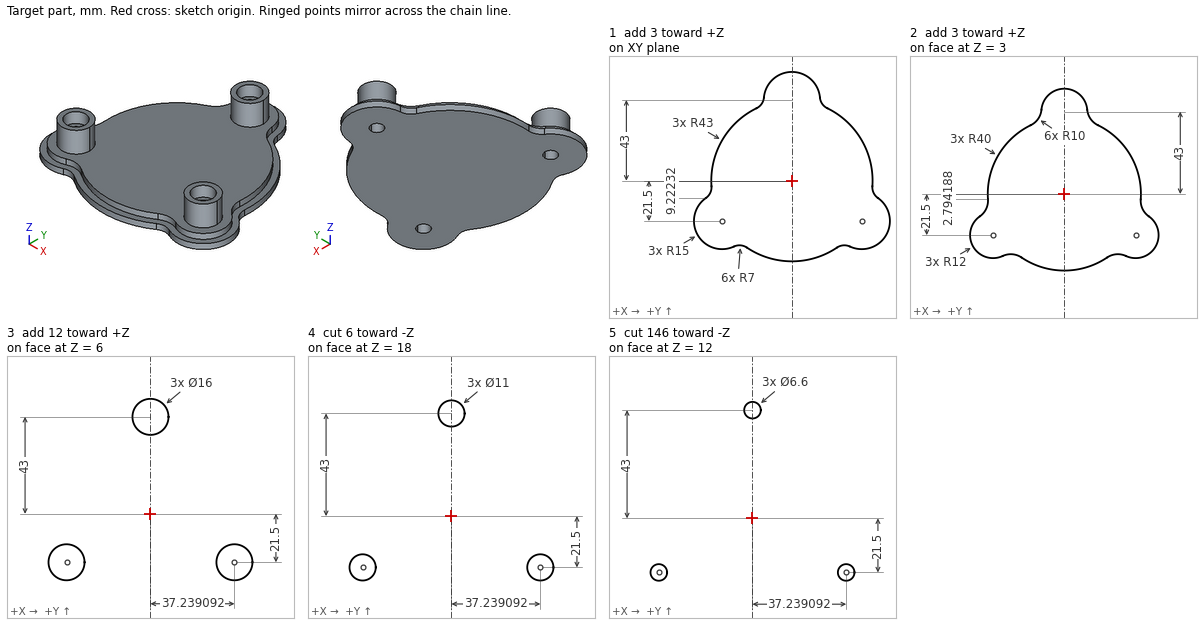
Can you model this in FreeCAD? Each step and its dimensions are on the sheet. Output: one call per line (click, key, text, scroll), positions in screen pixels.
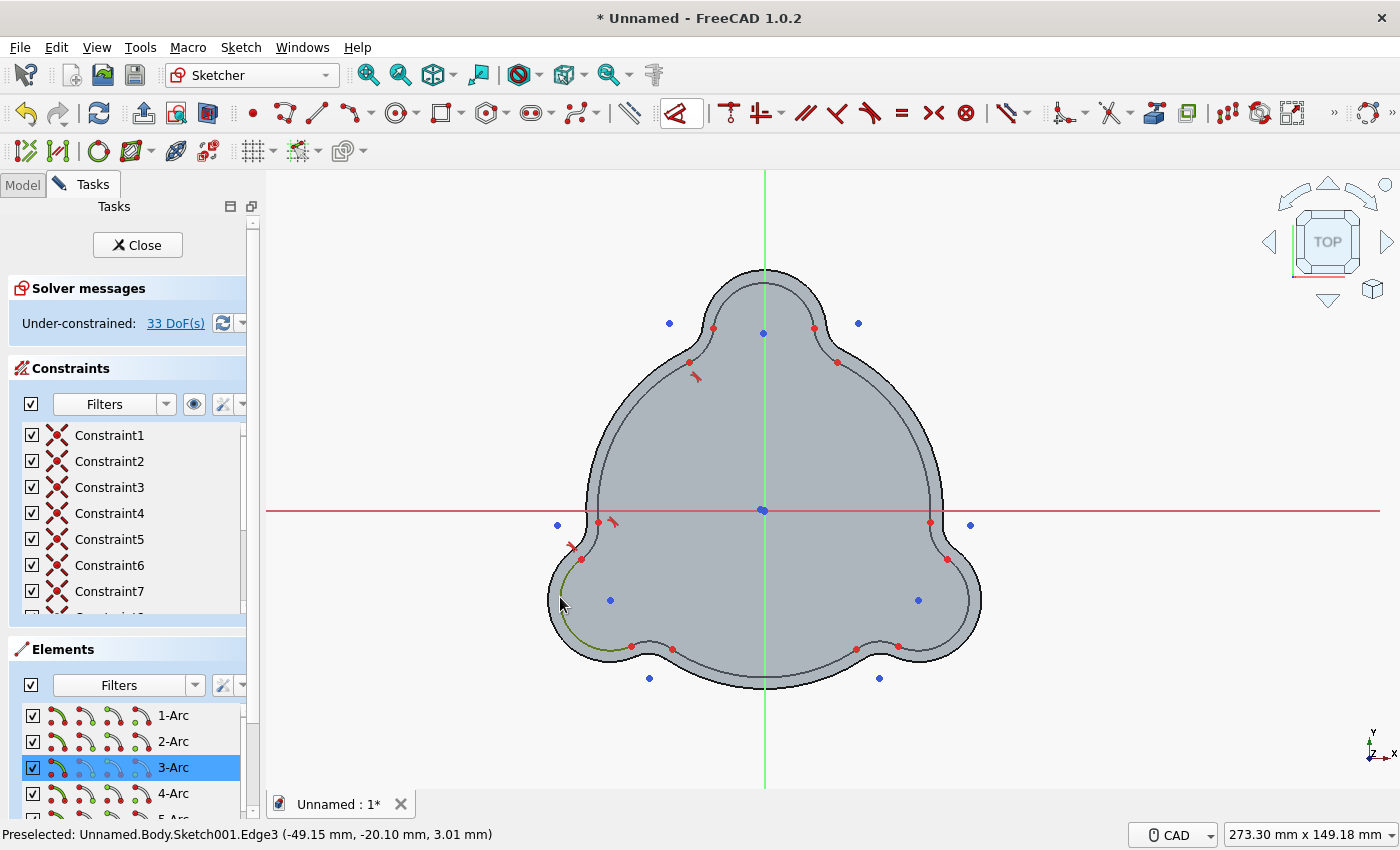
click(661, 643)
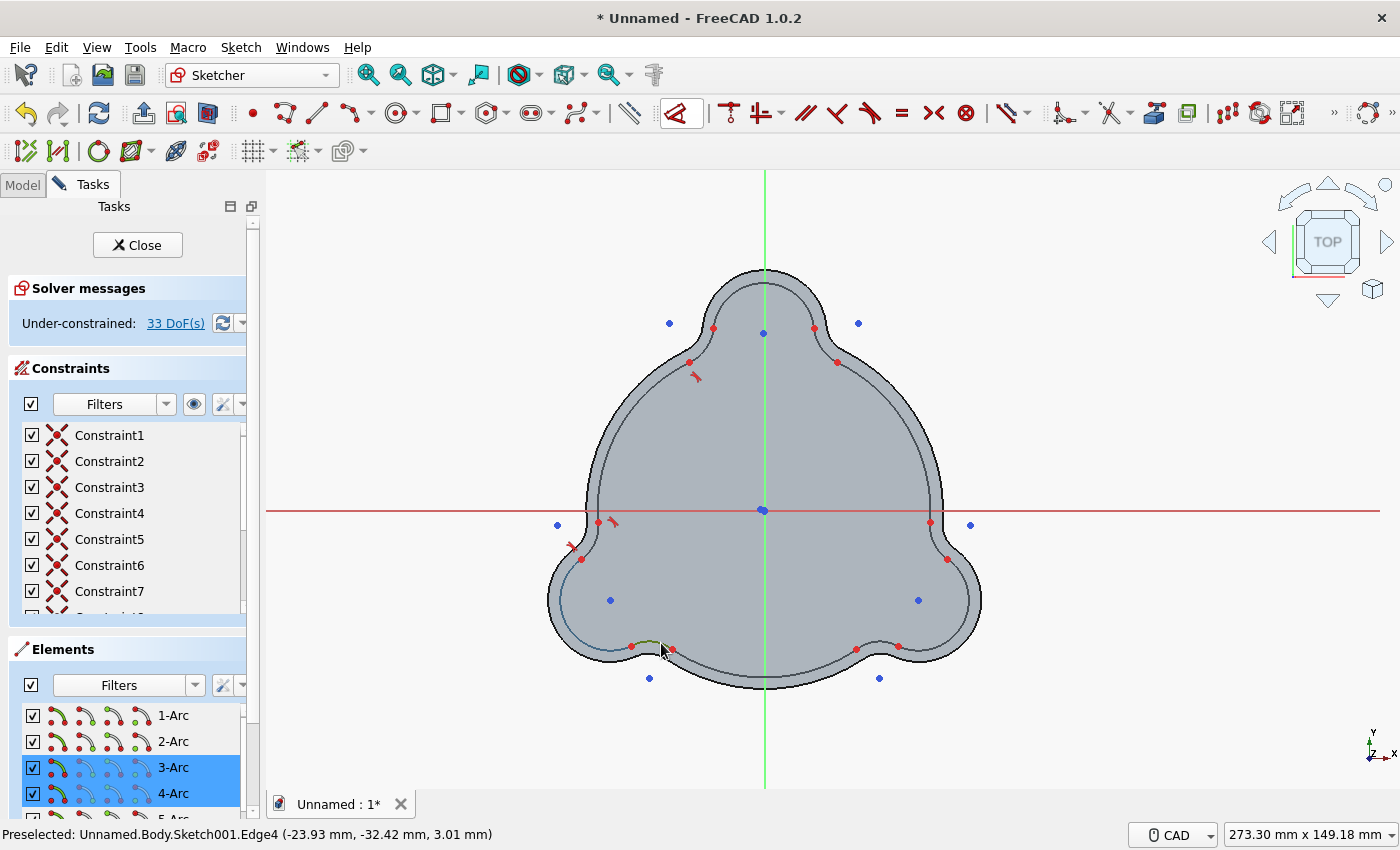
click(870, 114)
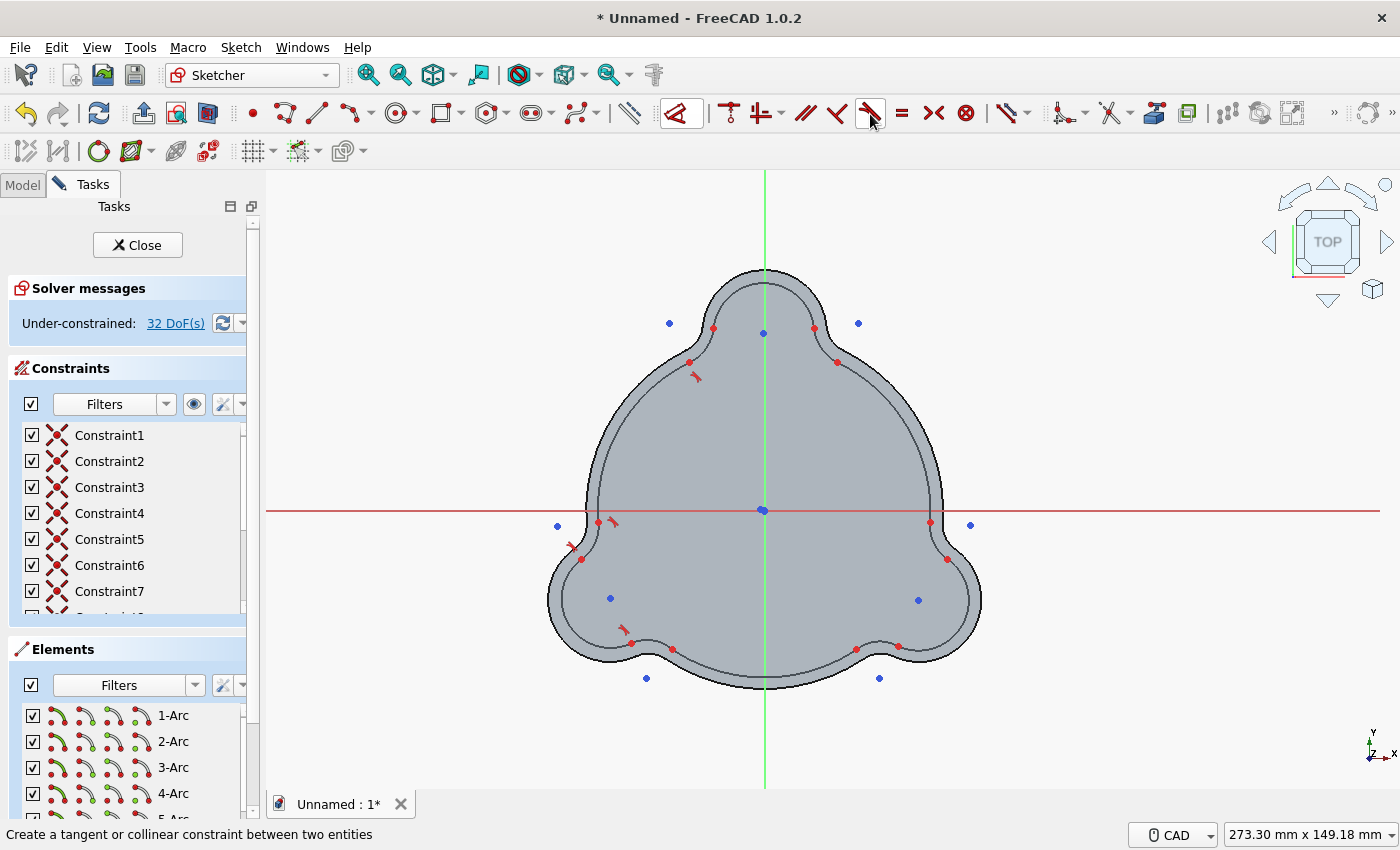
click(661, 643)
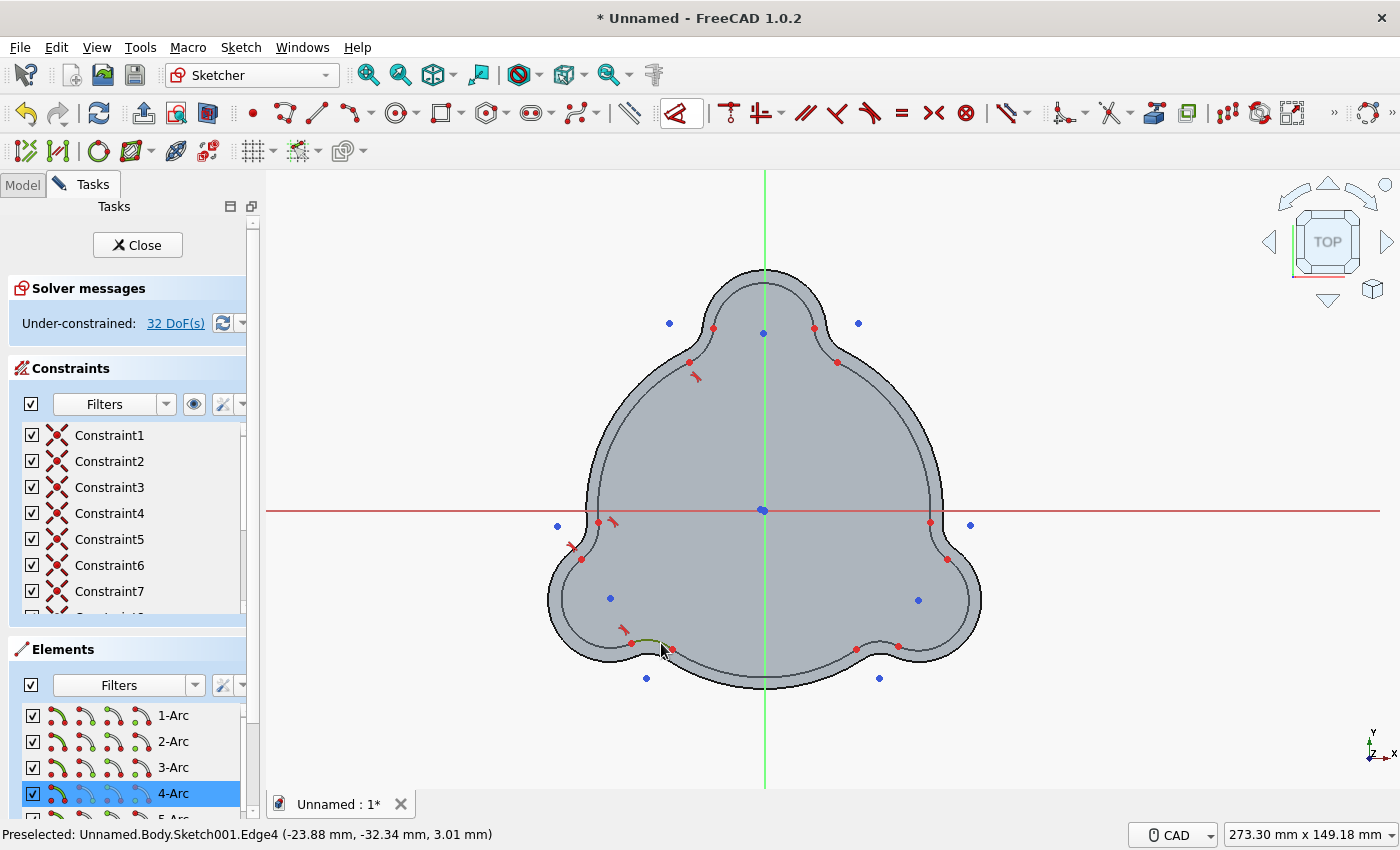
click(726, 673)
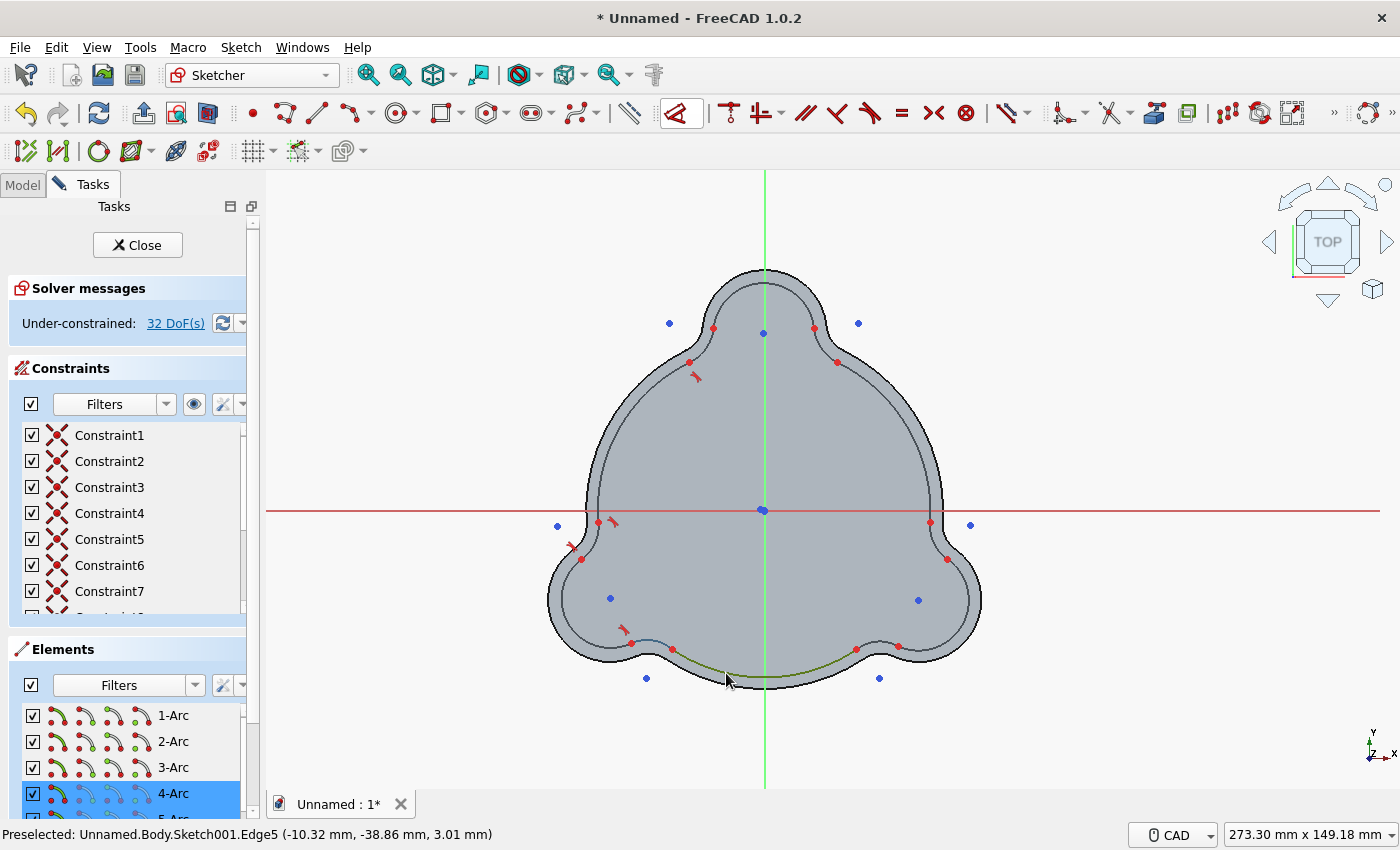
click(870, 114)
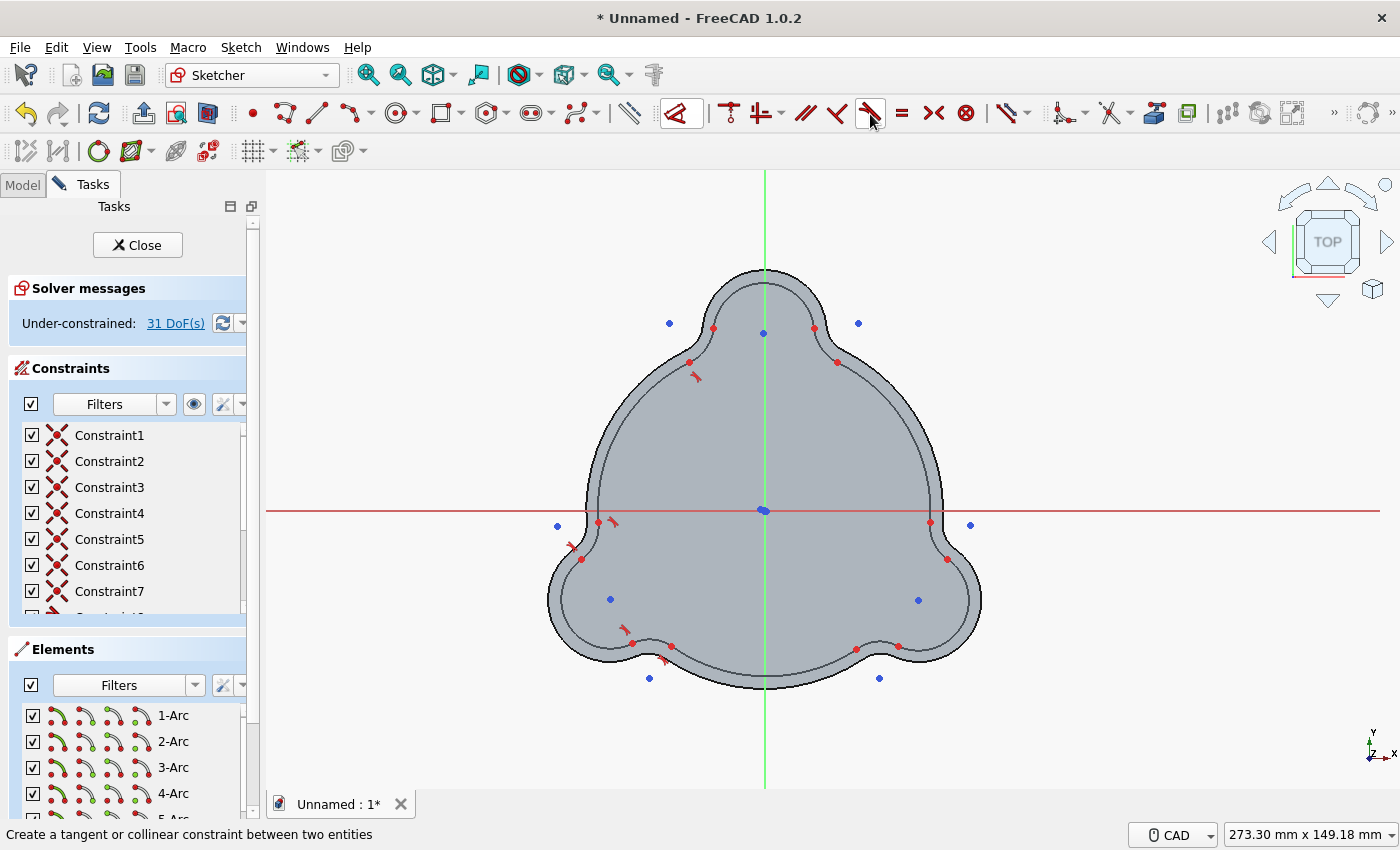
click(725, 671)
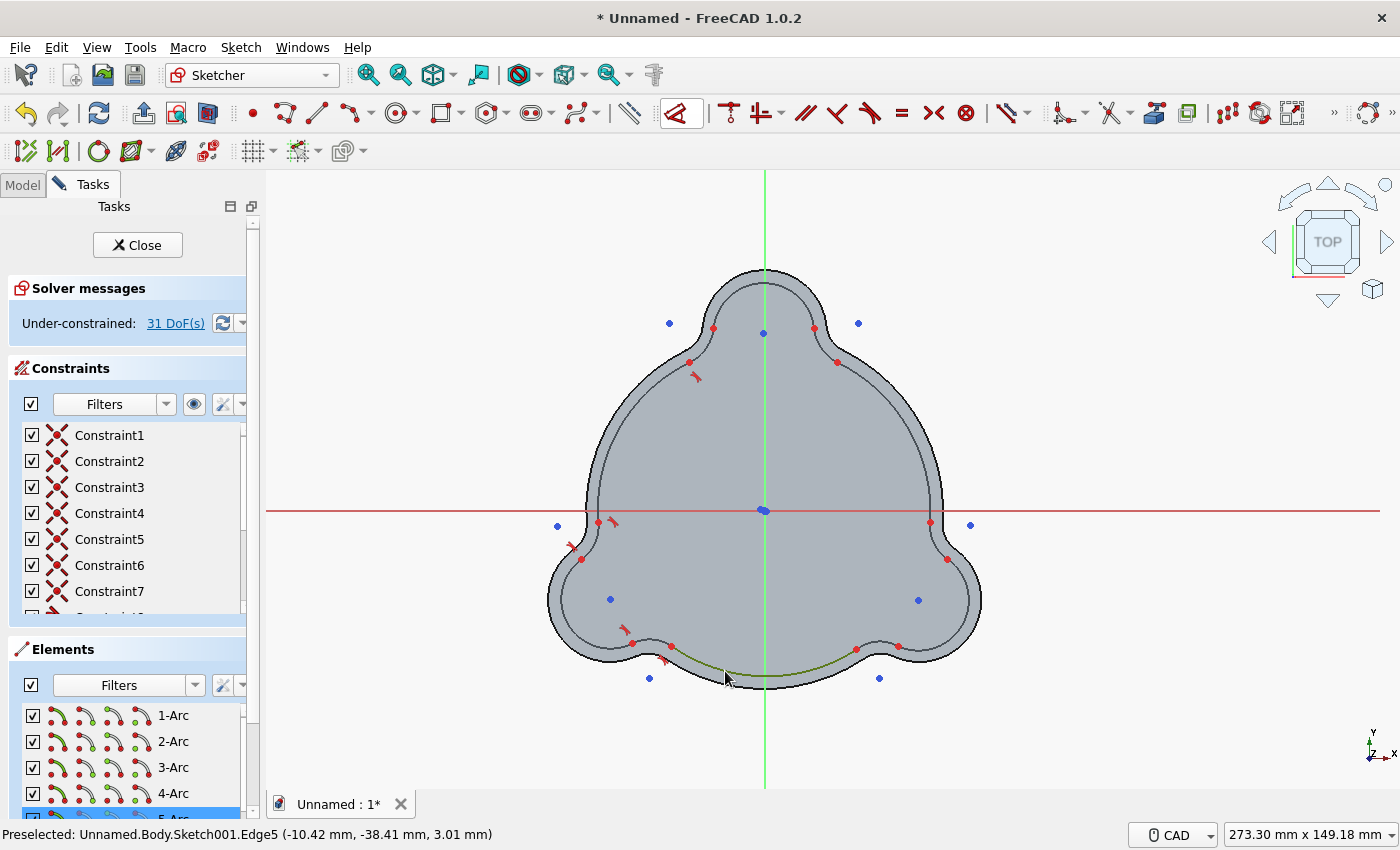
click(886, 642)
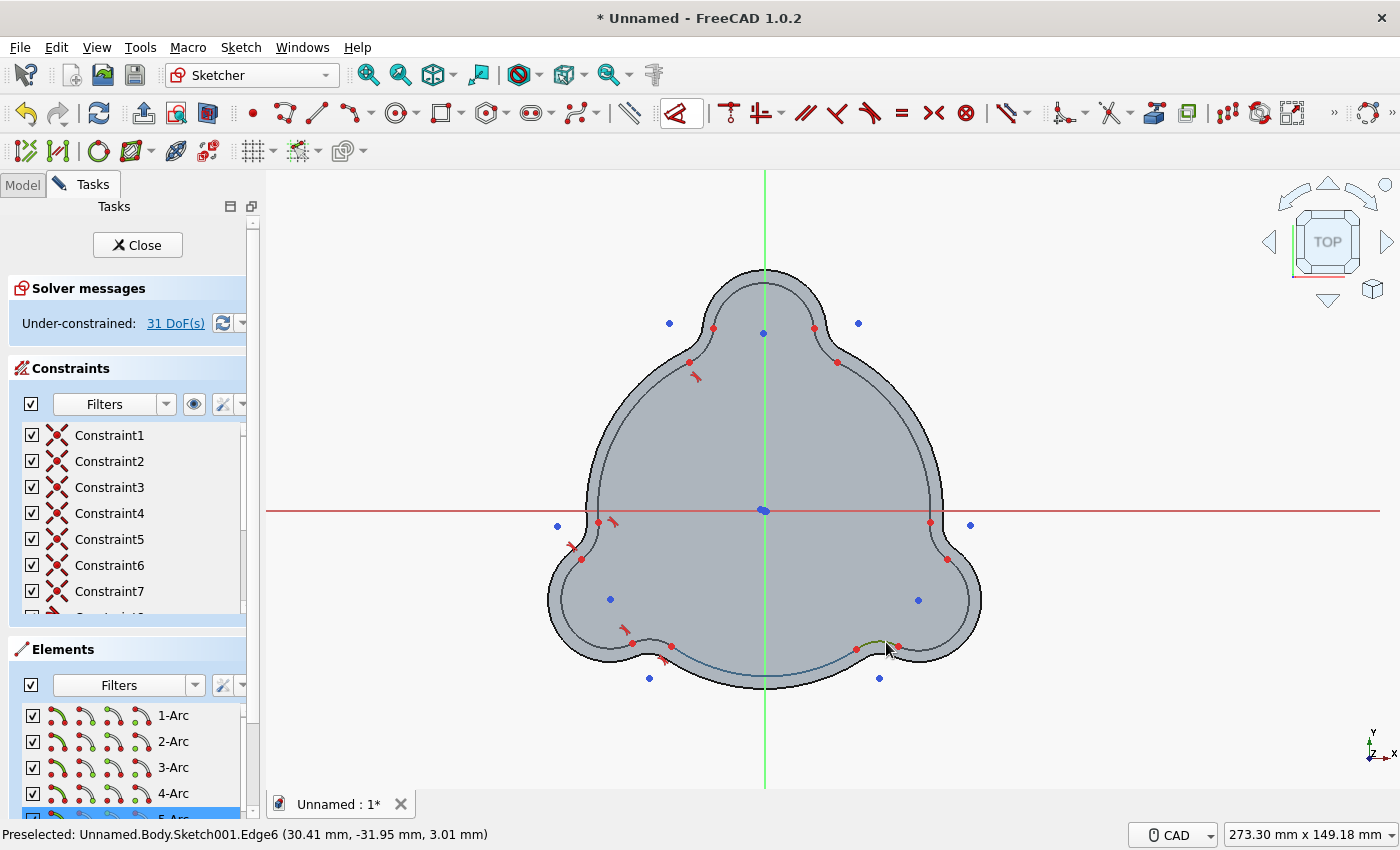
click(870, 114)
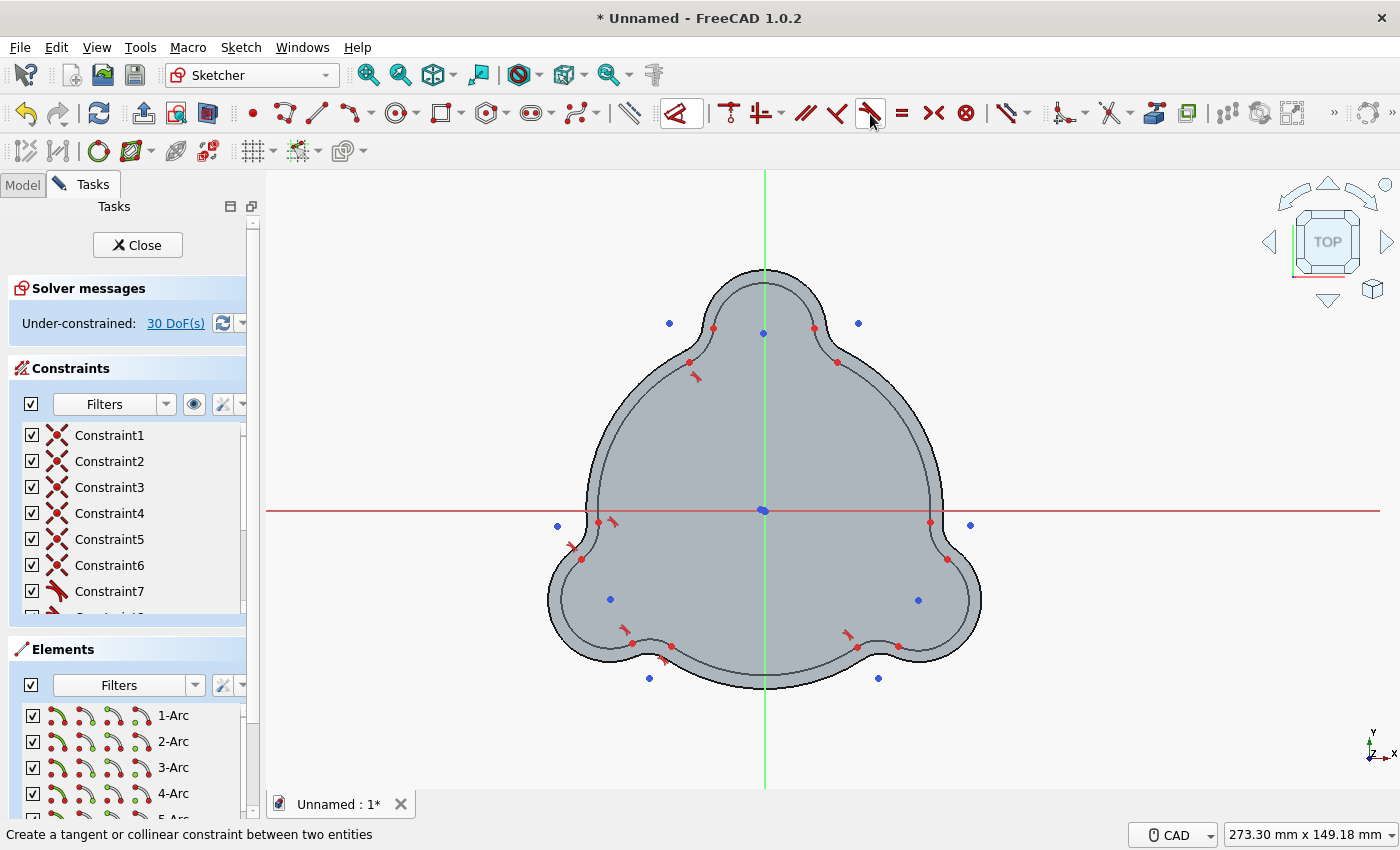
click(886, 641)